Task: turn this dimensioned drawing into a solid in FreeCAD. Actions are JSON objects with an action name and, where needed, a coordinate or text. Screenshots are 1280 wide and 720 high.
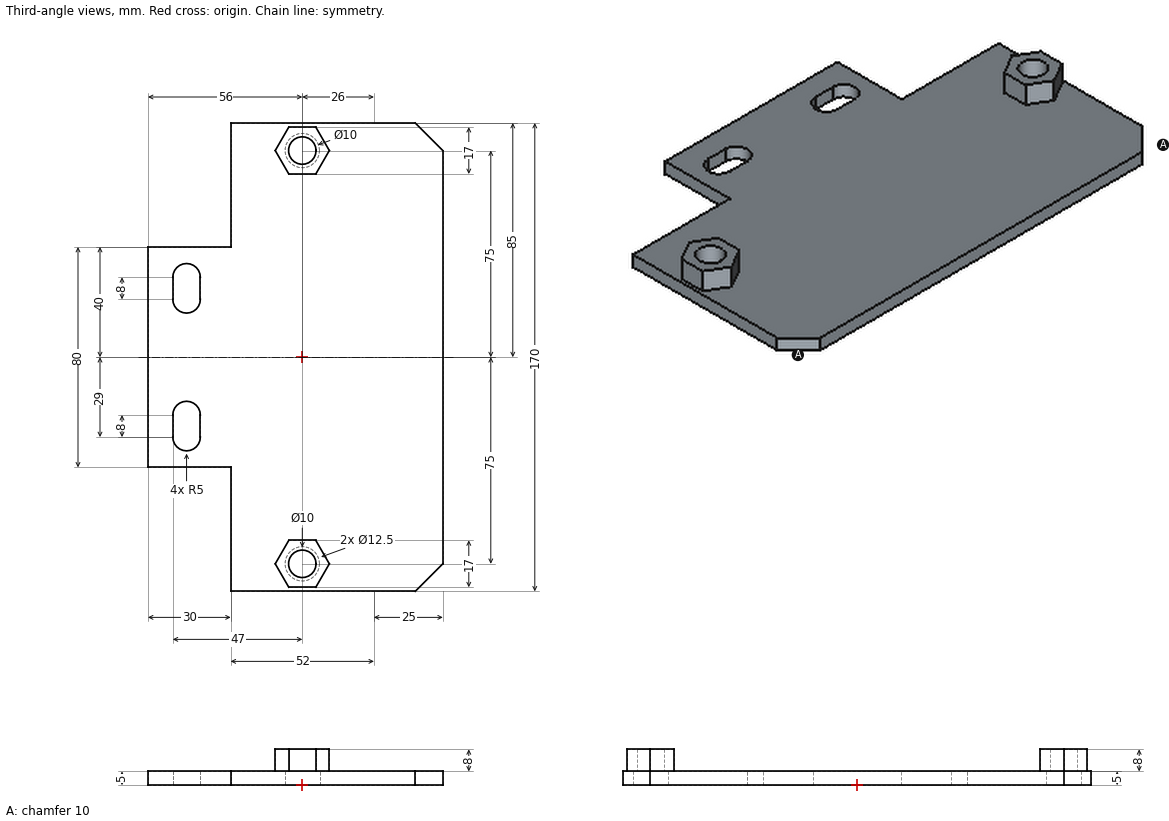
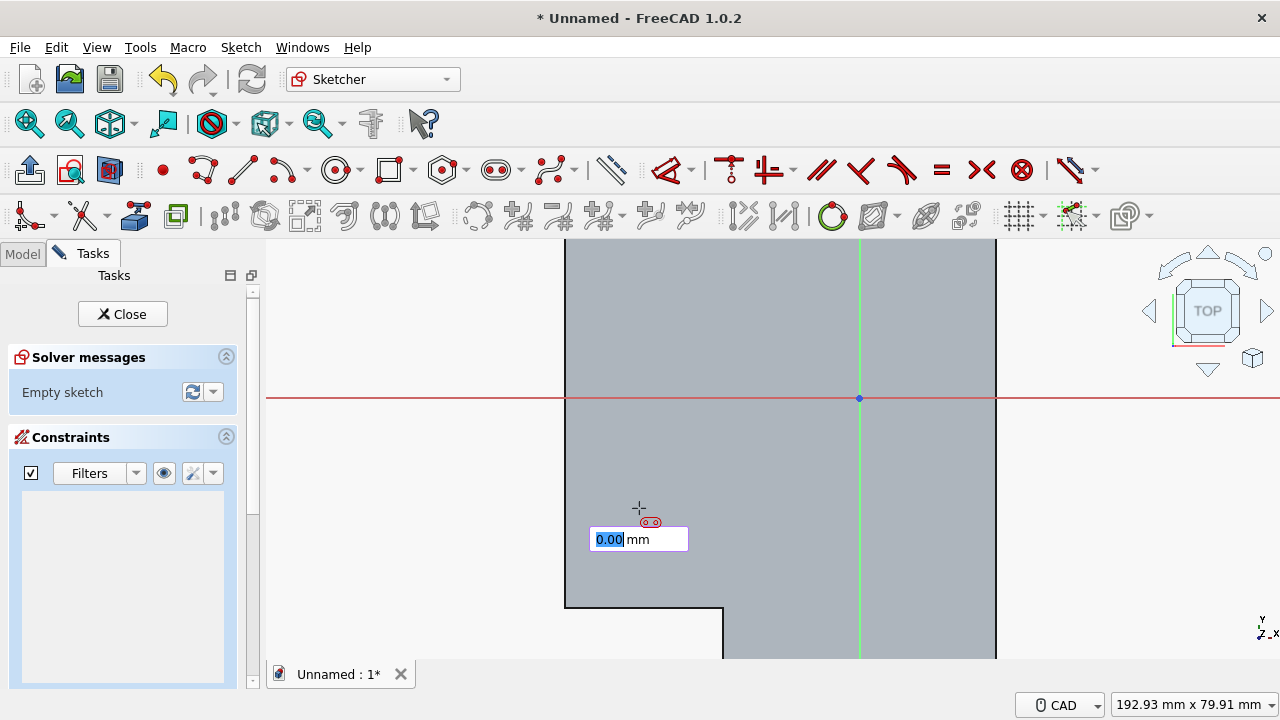
{"action": "left_click", "coordinate": [613, 529]}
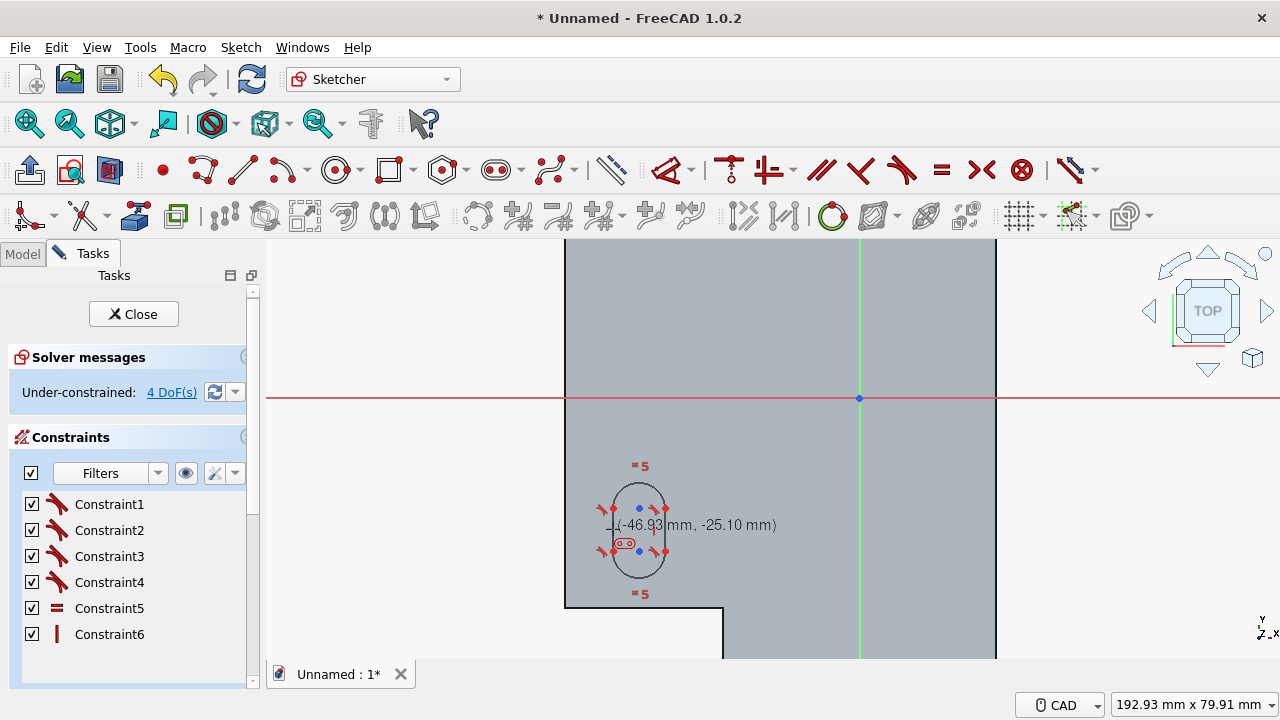
{"action": "left_click", "coordinate": [639, 288]}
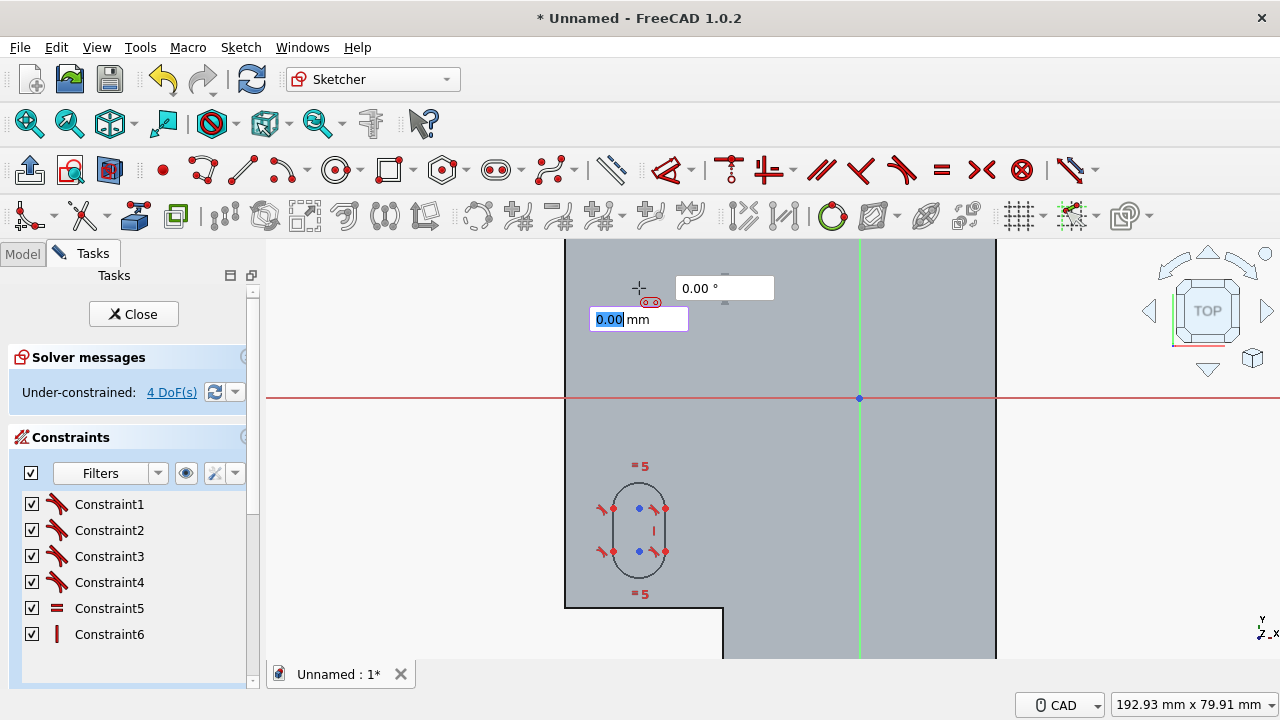
{"action": "scroll", "coordinate": [640, 552], "scroll_direction": "down", "scroll_amount": 2}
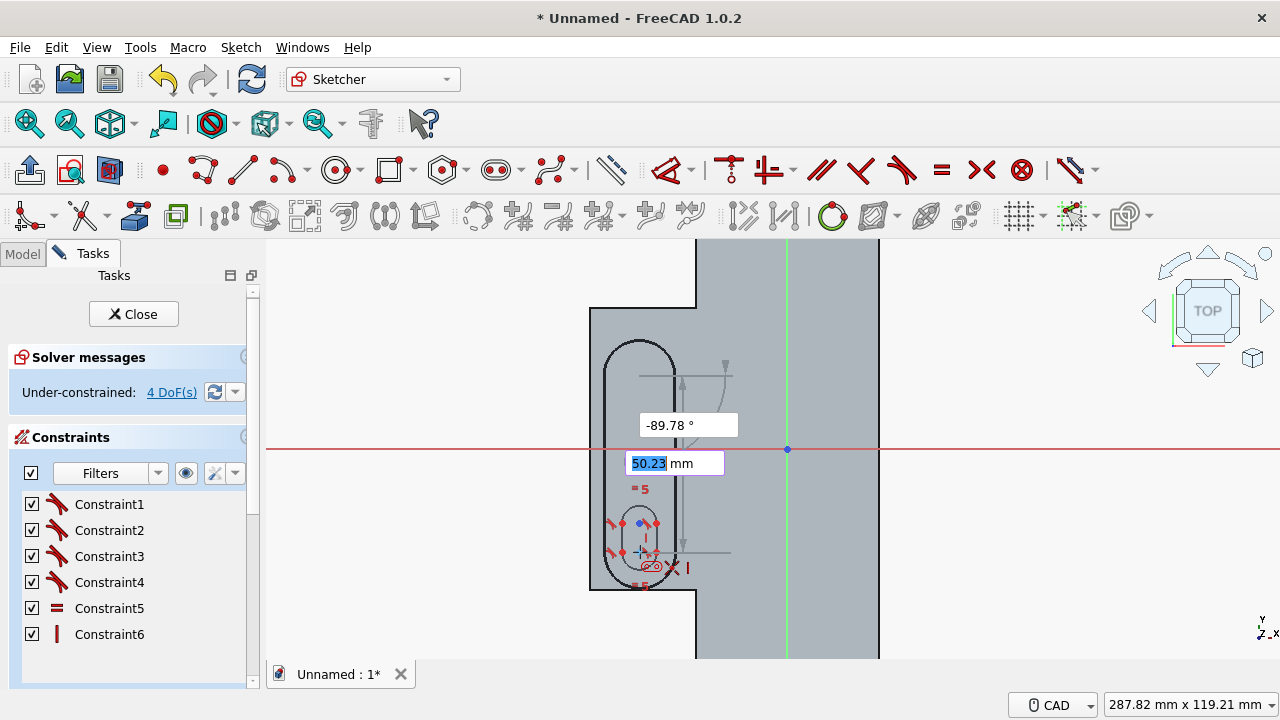
{"action": "left_click", "coordinate": [639, 347]}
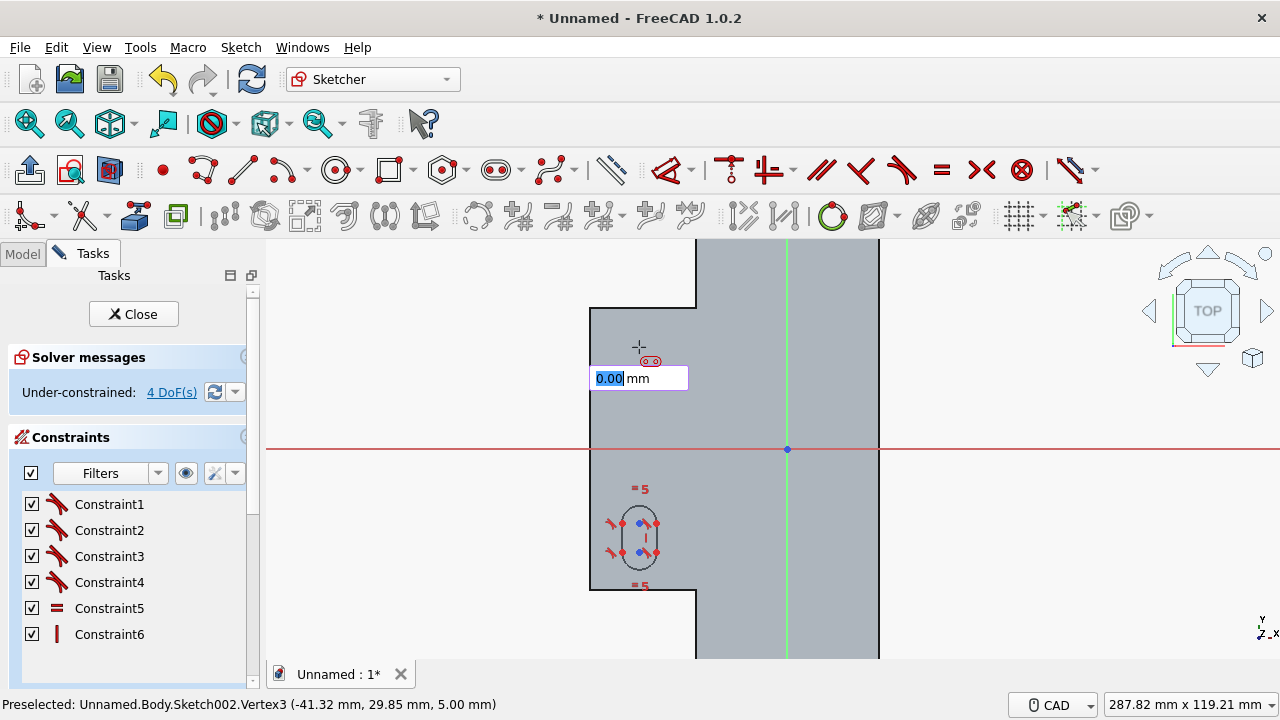
{"action": "left_click", "coordinate": [622, 361]}
{"action": "key", "text": "Escape"}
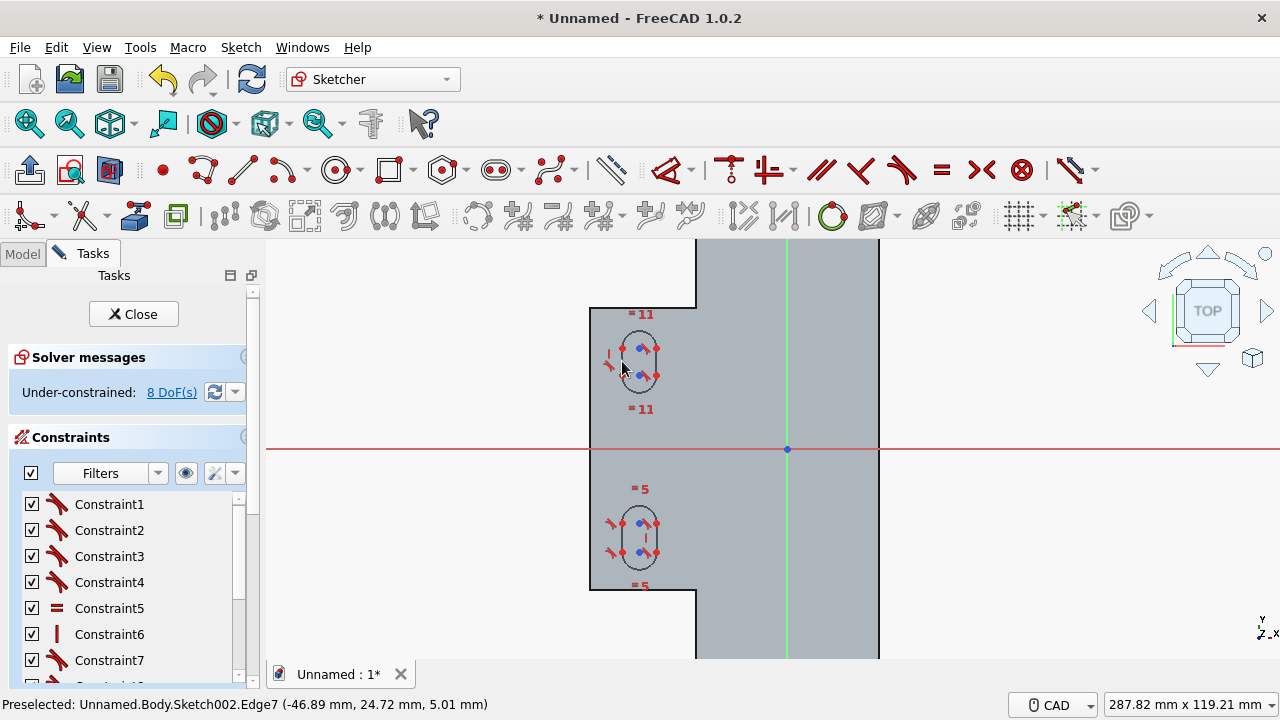
{"action": "left_click", "coordinate": [629, 566]}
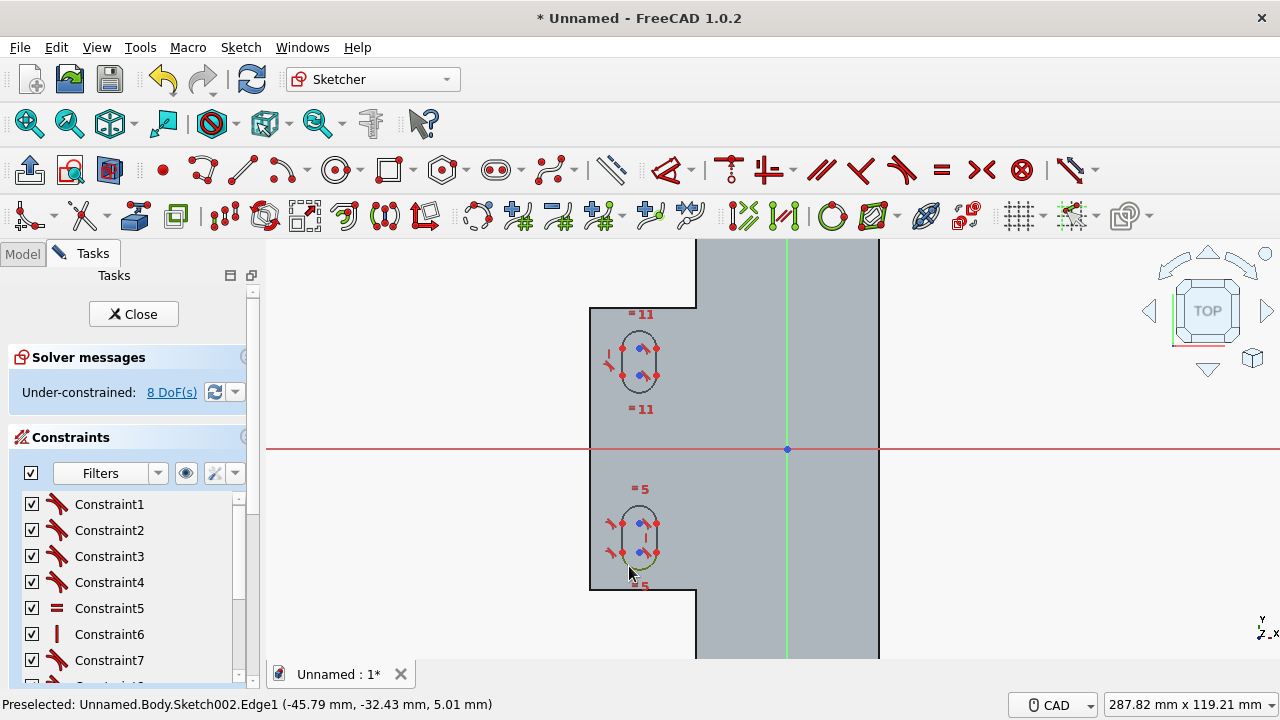
{"action": "left_click", "coordinate": [629, 390]}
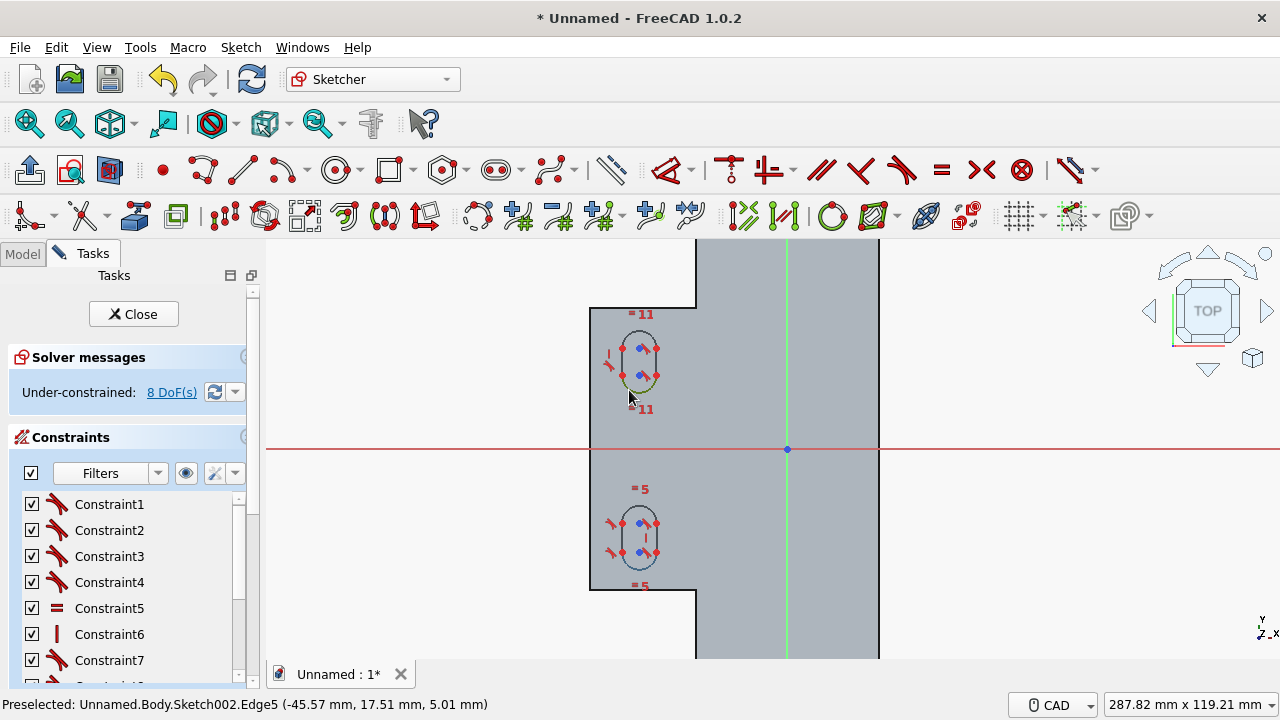
{"action": "left_click", "coordinate": [942, 170]}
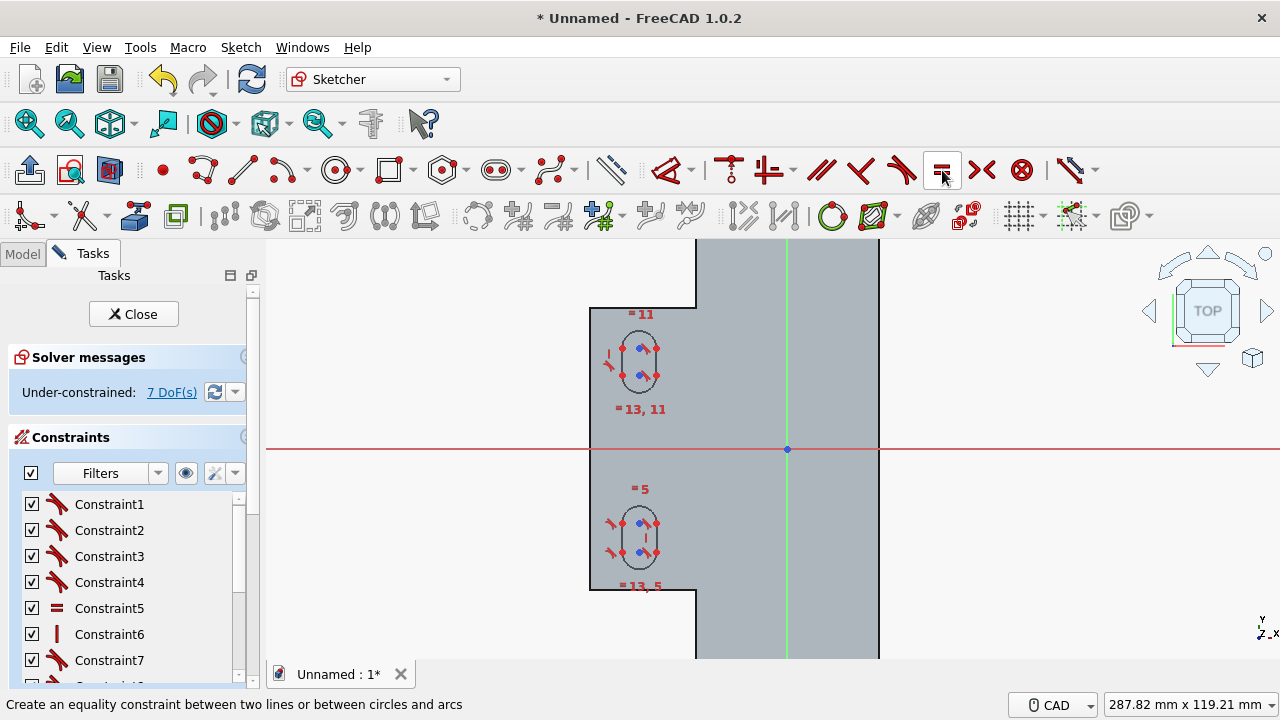
{"action": "left_click", "coordinate": [639, 523]}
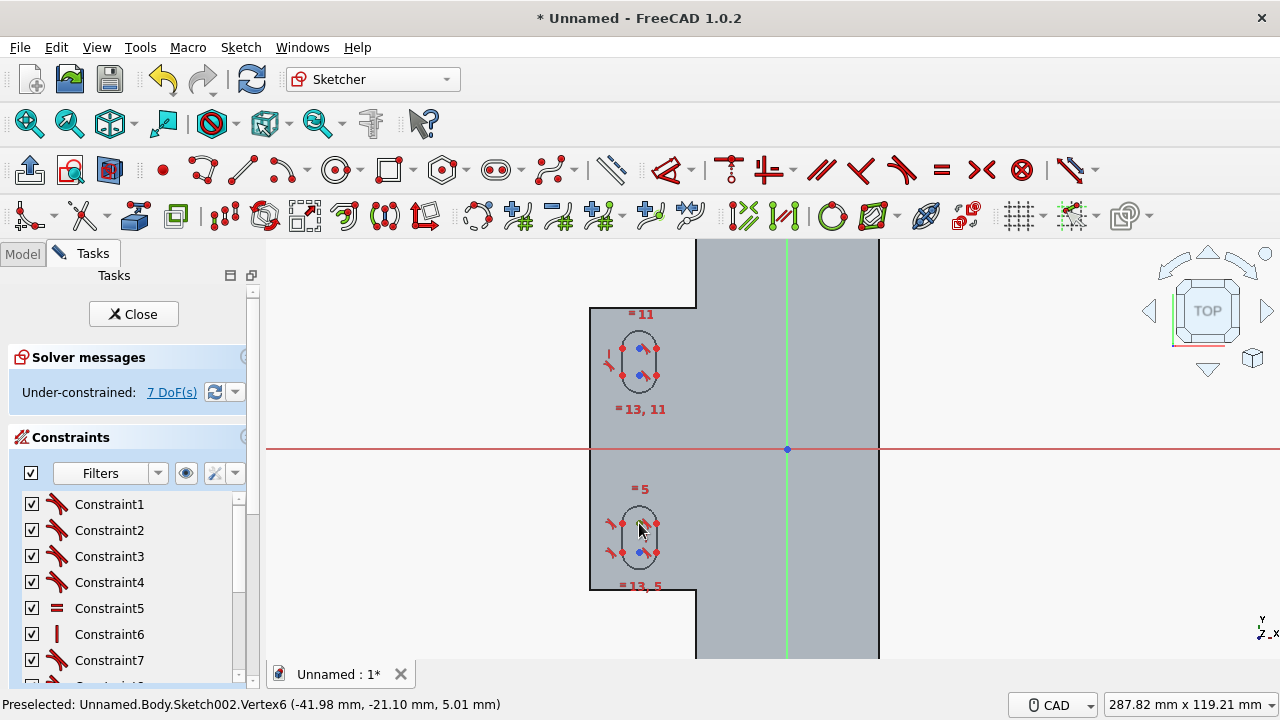
{"action": "left_click", "coordinate": [639, 376]}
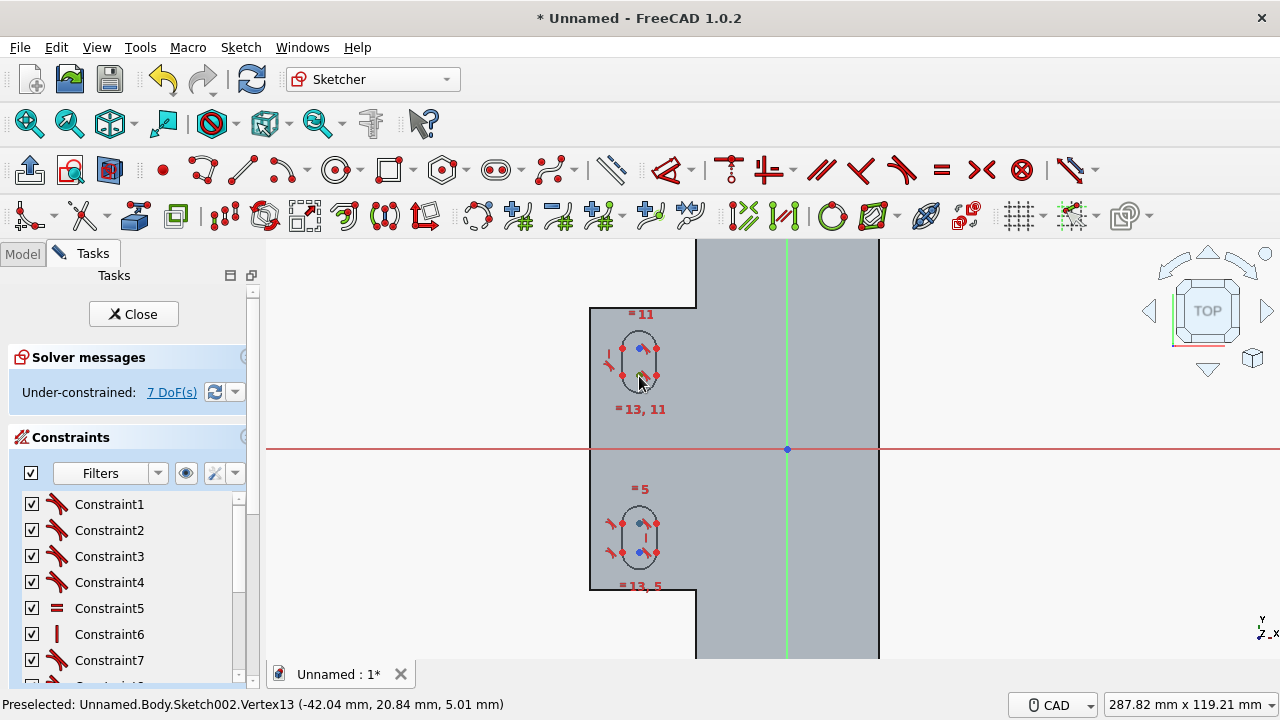
{"action": "left_click", "coordinate": [353, 449]}